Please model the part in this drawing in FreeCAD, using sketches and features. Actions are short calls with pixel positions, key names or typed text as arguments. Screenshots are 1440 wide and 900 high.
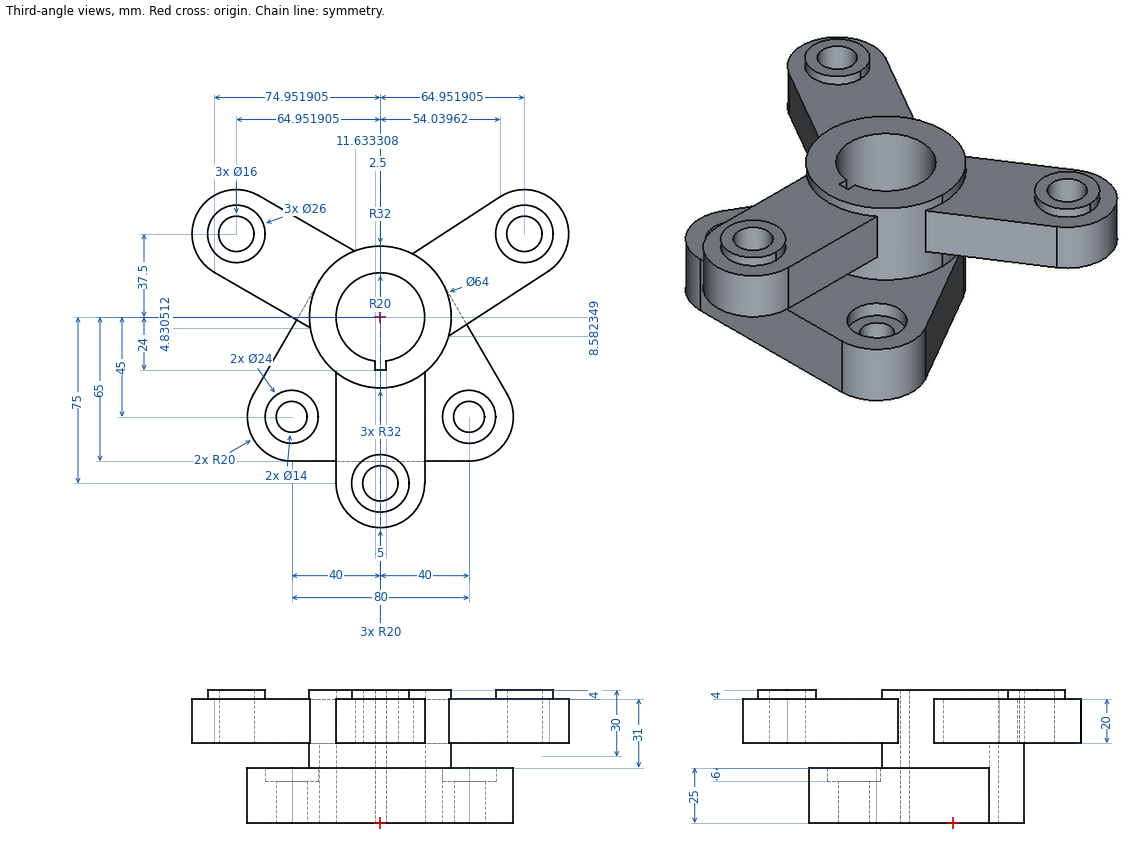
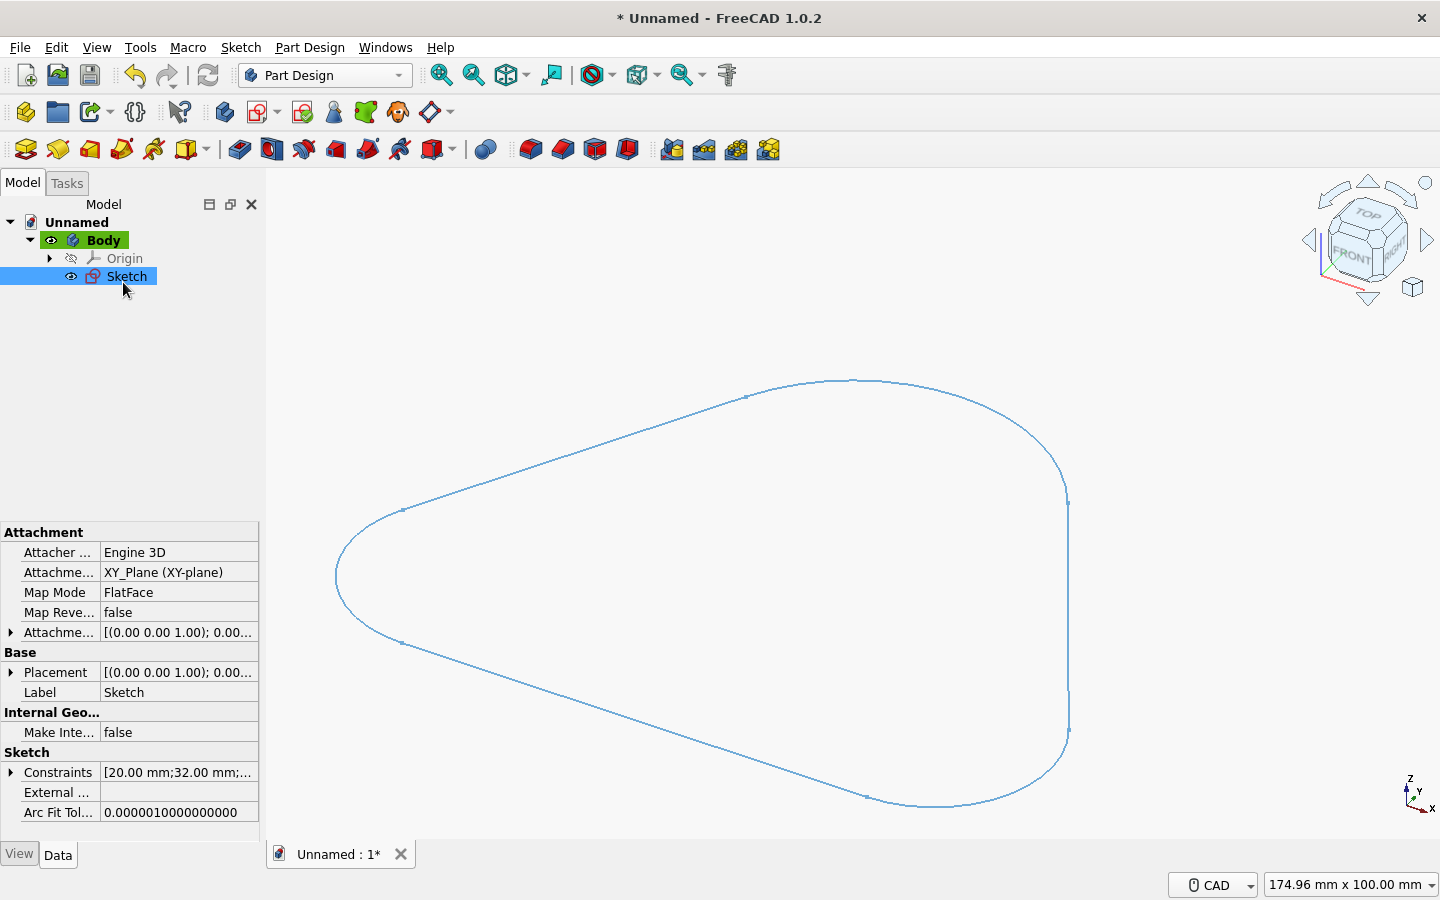
click(26, 150)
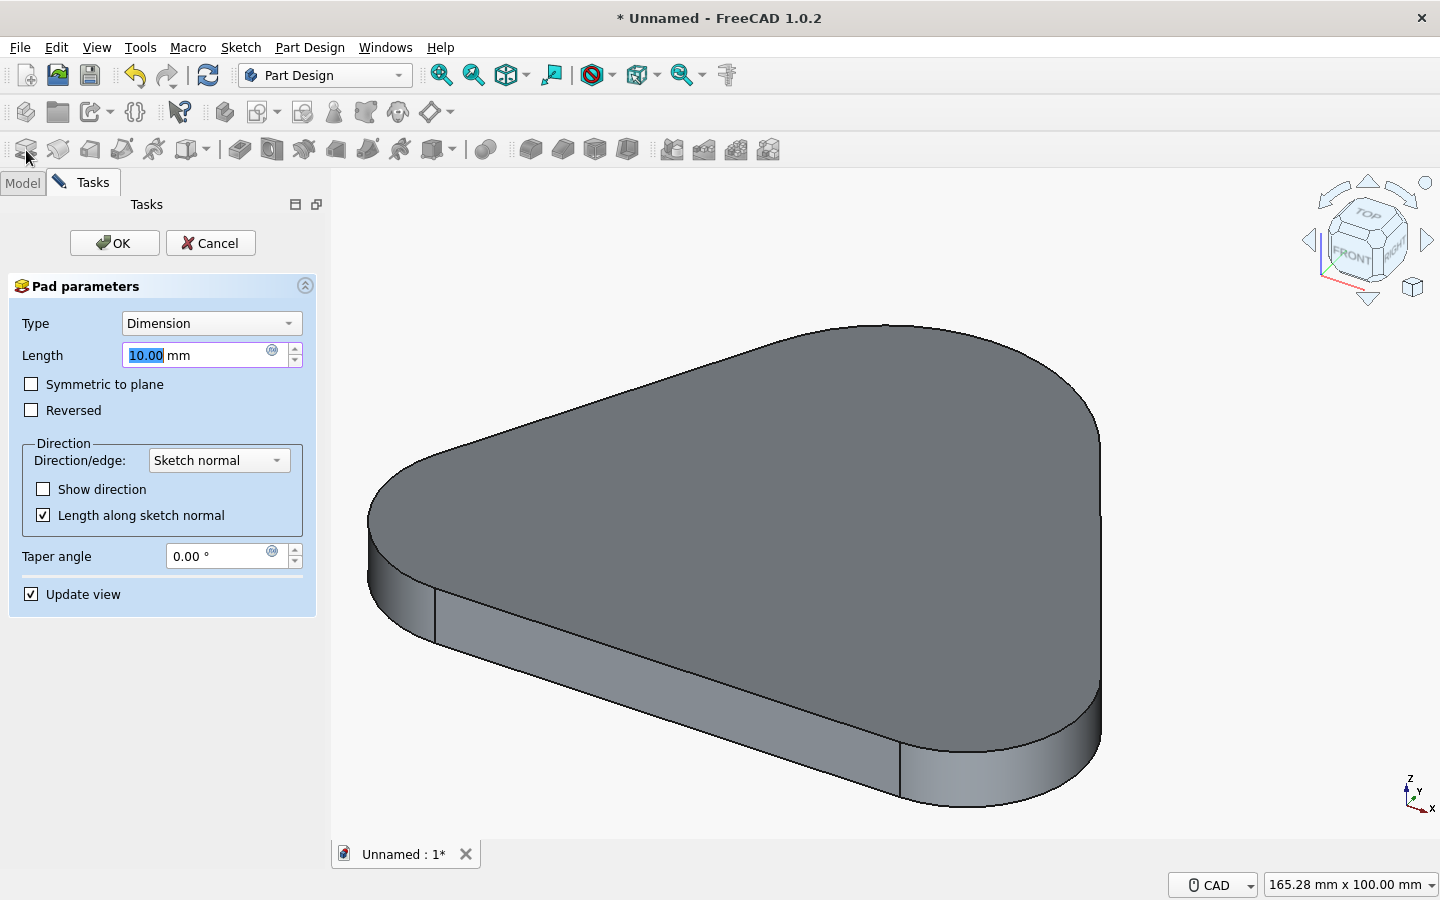
text(25)
key(Tab)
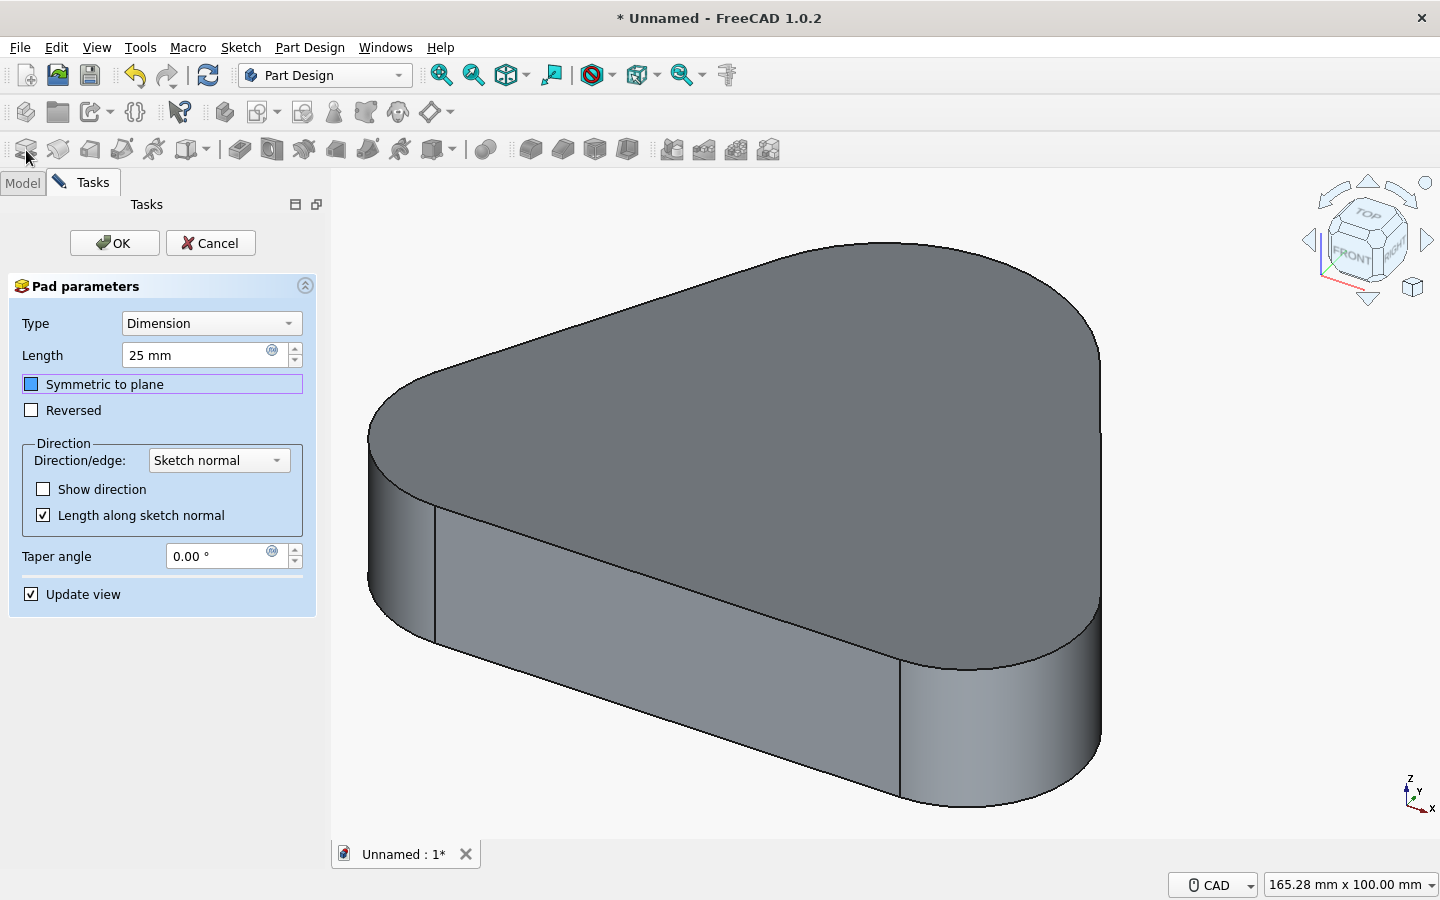
click(115, 243)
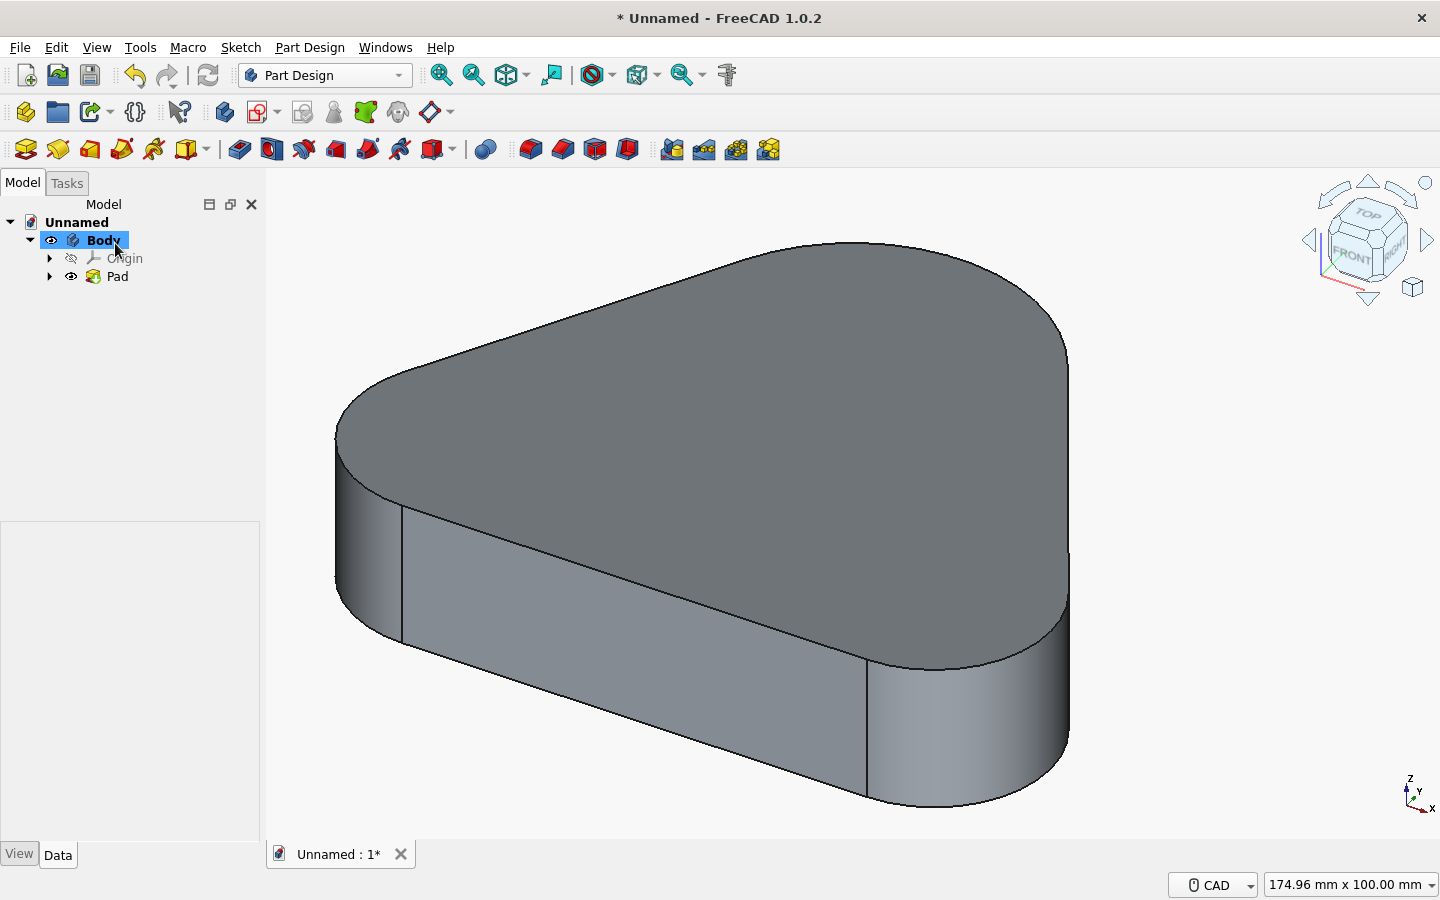
click(442, 76)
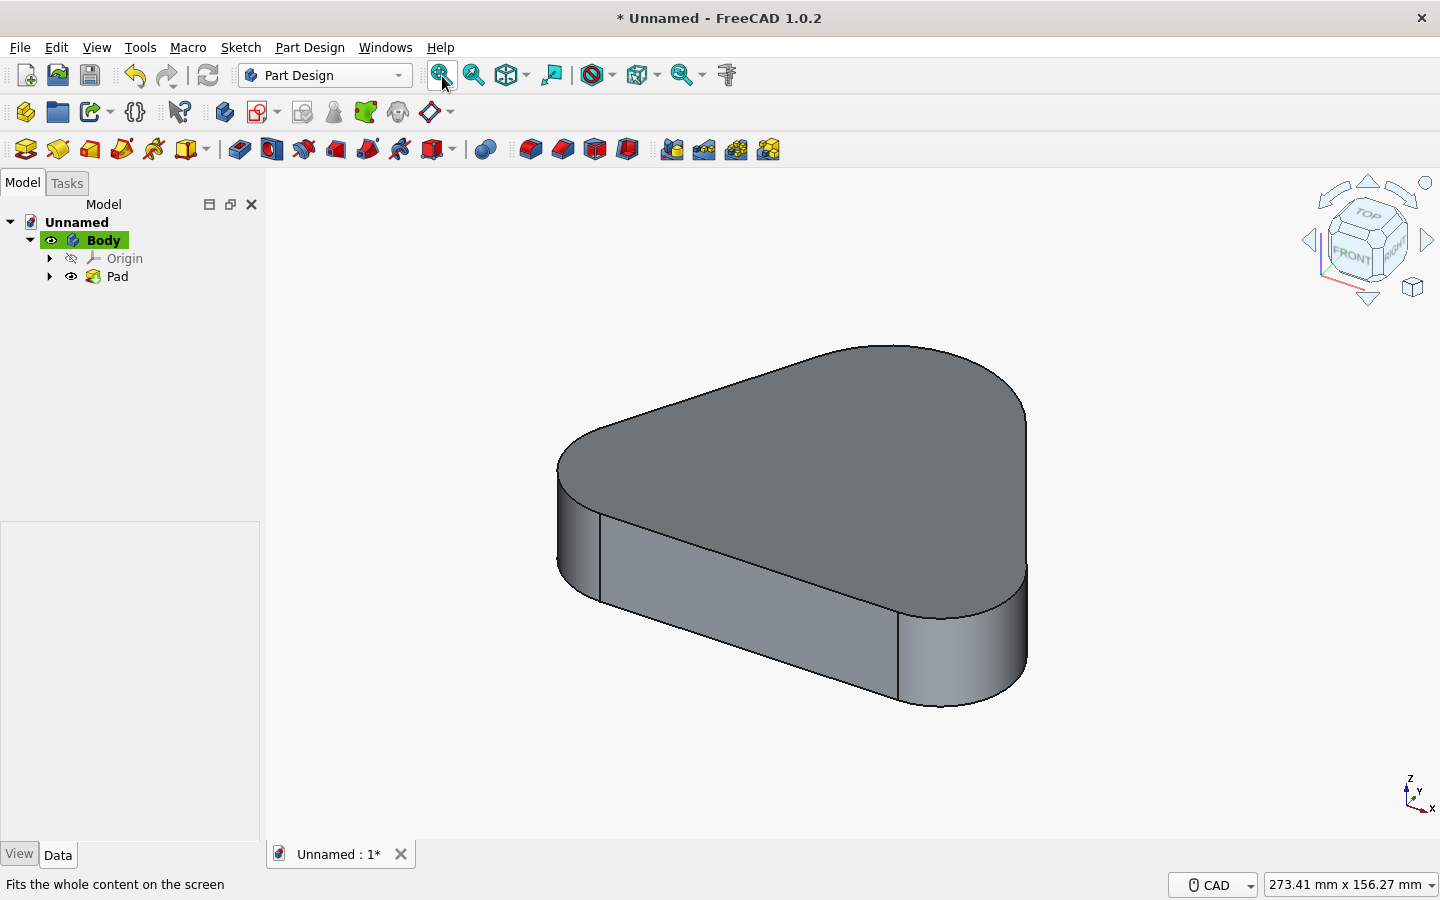
click(853, 458)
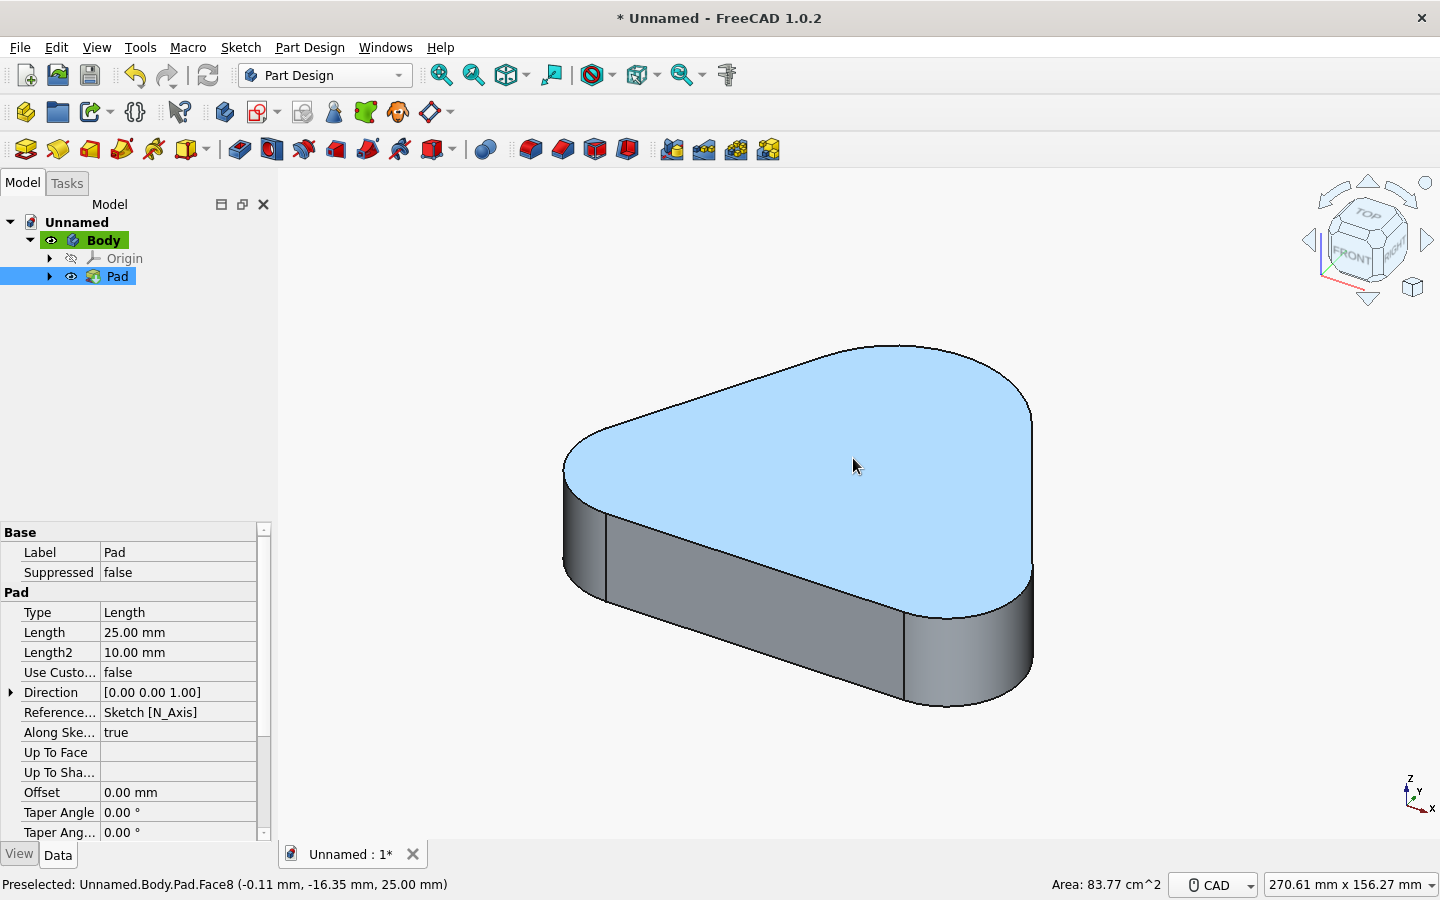
click(258, 112)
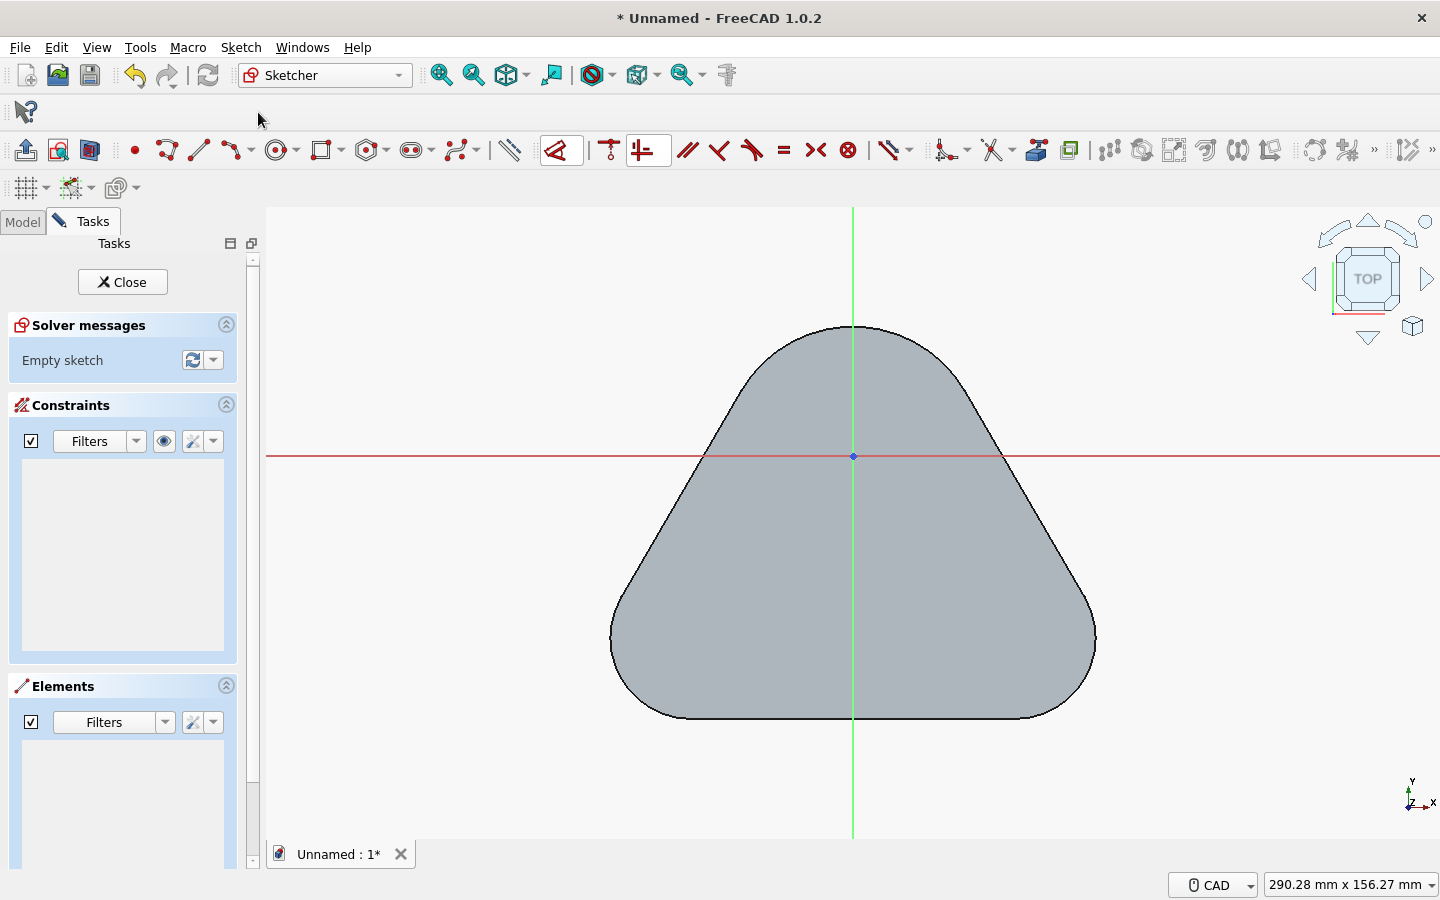
scroll(992, 320, up, 2)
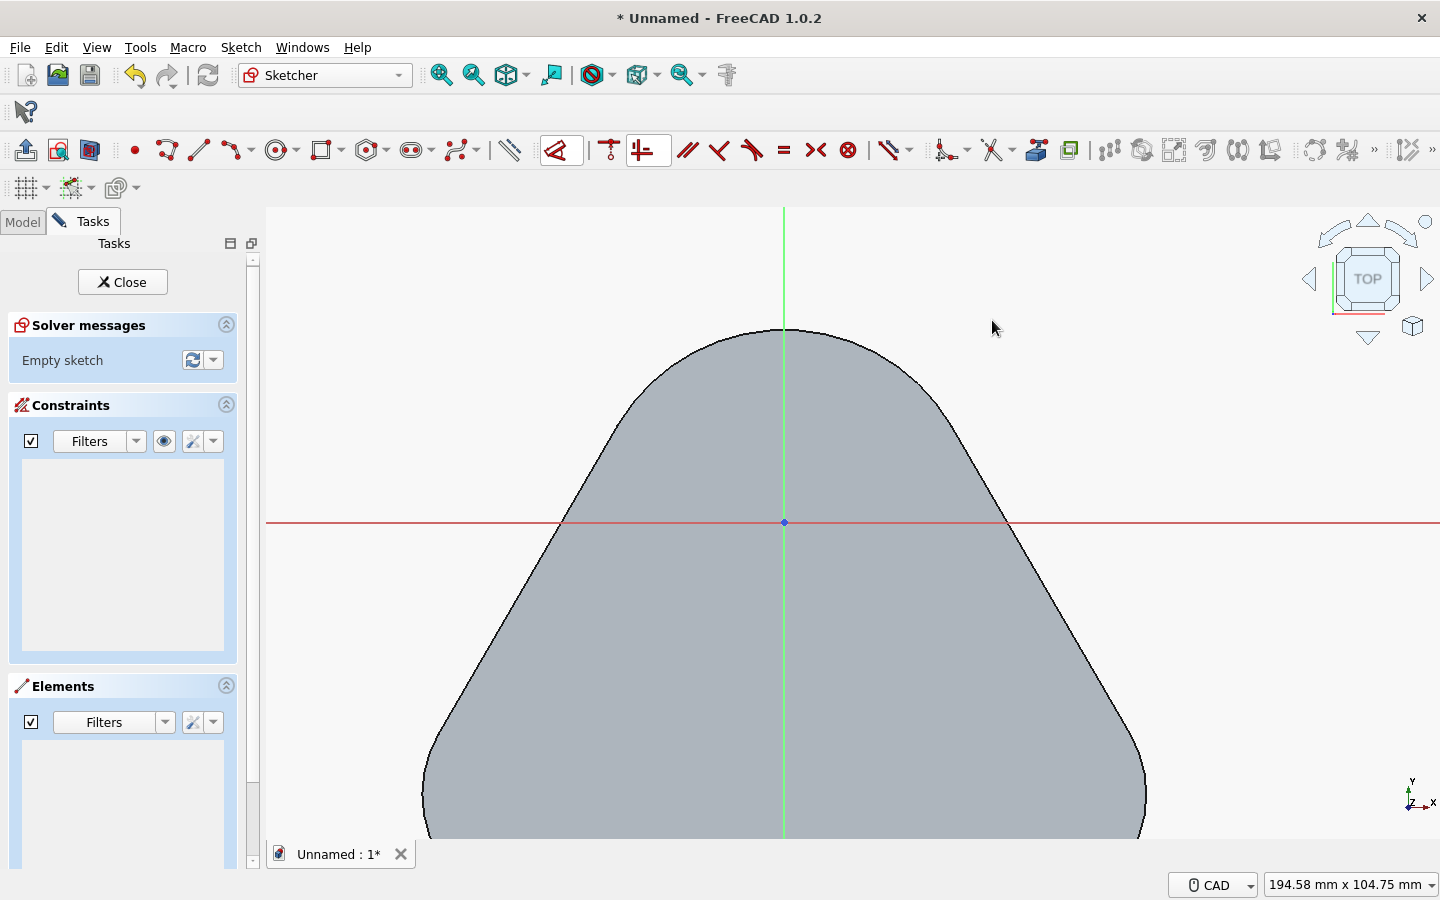
click(276, 150)